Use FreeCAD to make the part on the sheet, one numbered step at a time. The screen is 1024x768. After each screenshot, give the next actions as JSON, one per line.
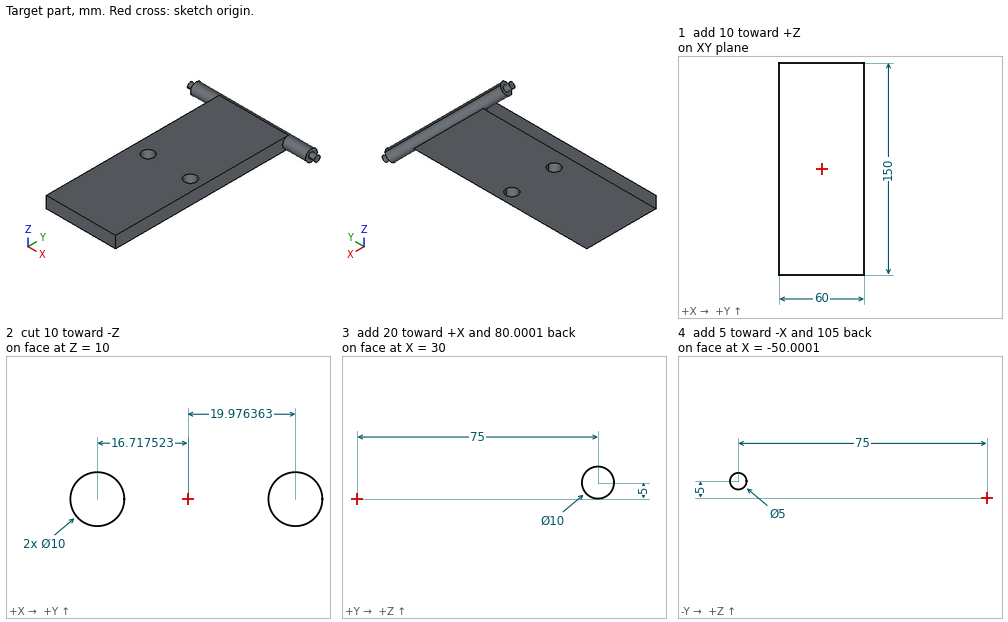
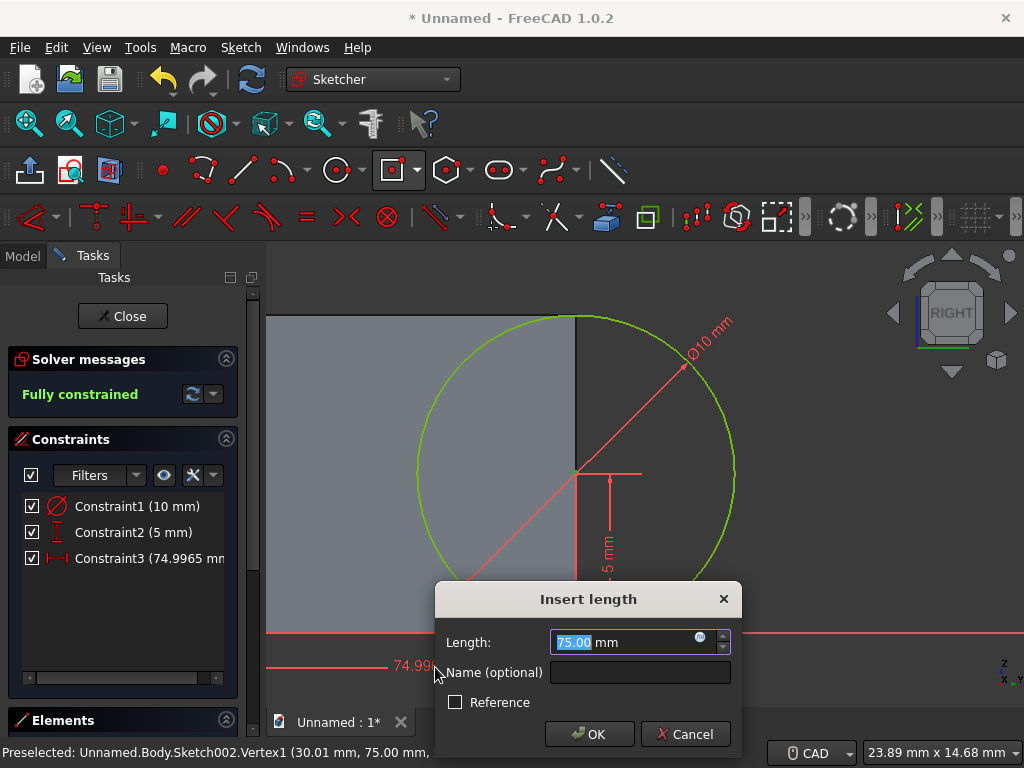
{"action": "type", "text": "75"}
{"action": "key", "text": "Return"}
{"action": "key", "text": "Escape"}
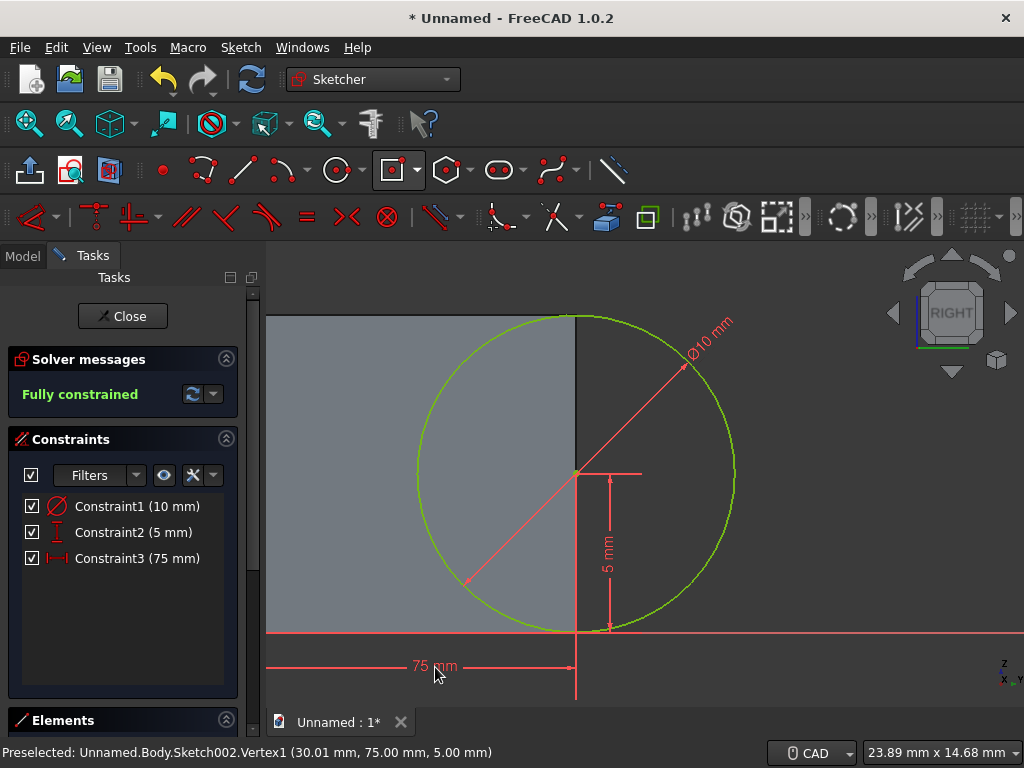
{"action": "left_click", "coordinate": [123, 316]}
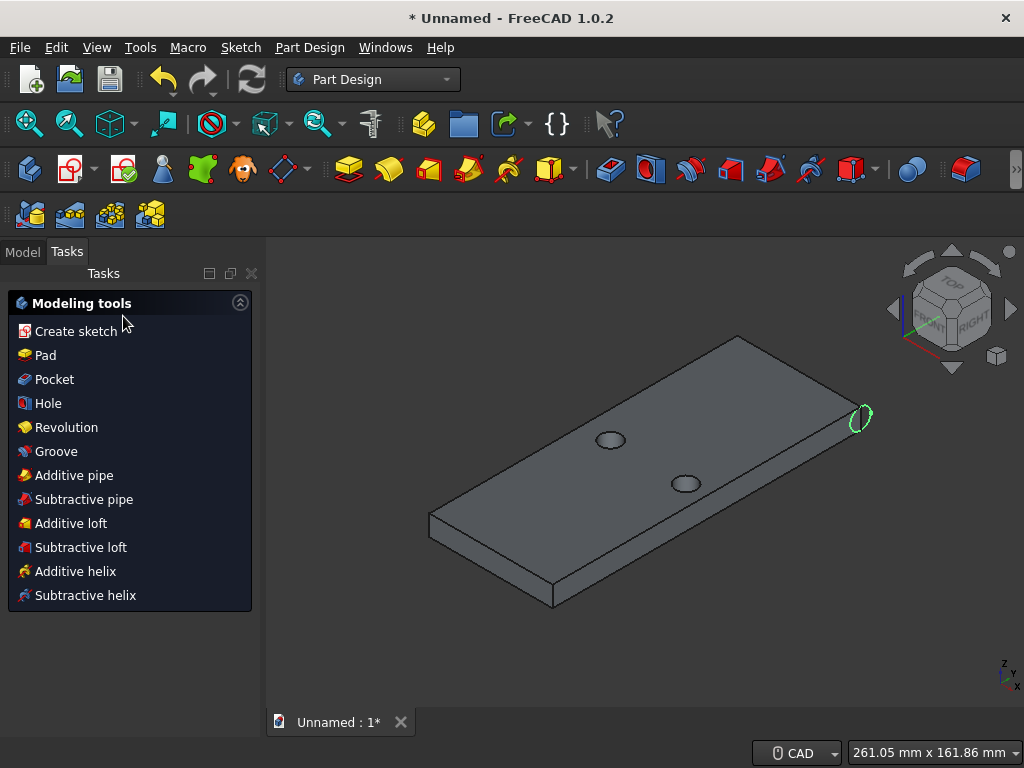
{"action": "left_click", "coordinate": [350, 170]}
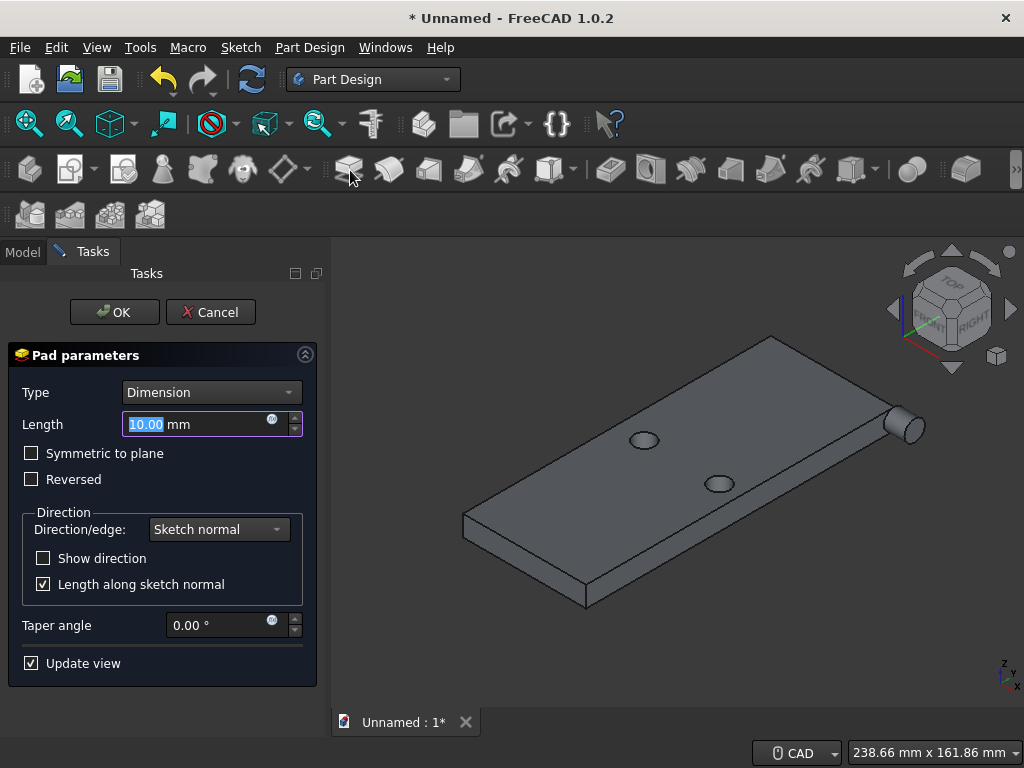
{"action": "left_click", "coordinate": [212, 392]}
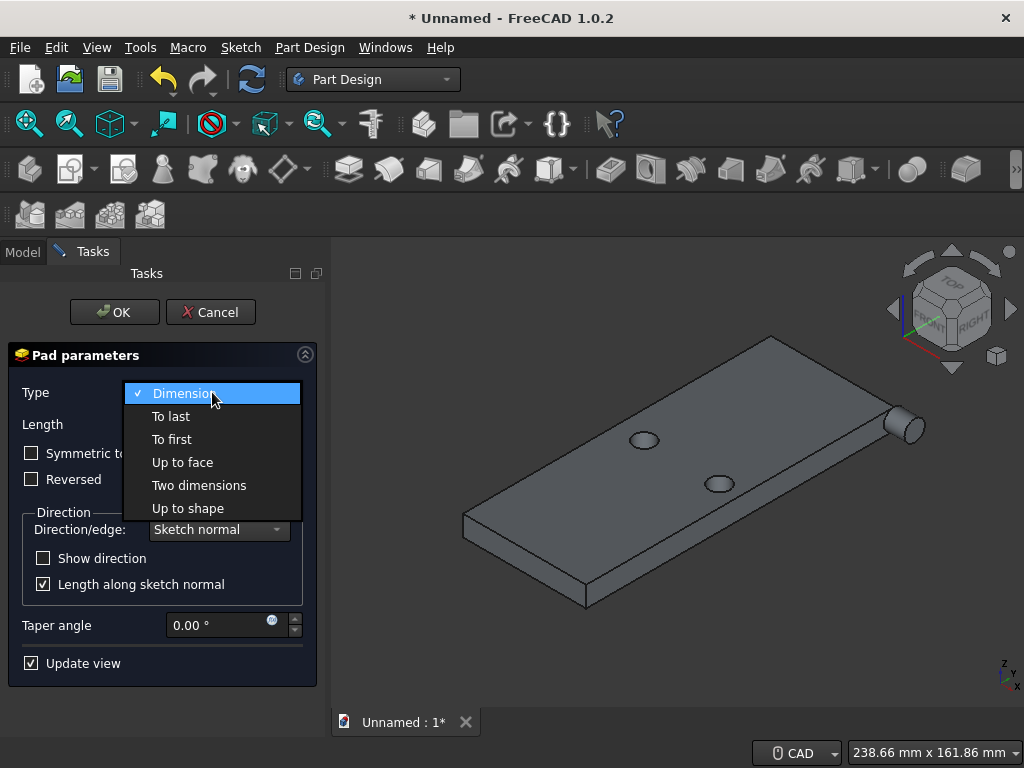
{"action": "left_click", "coordinate": [212, 486]}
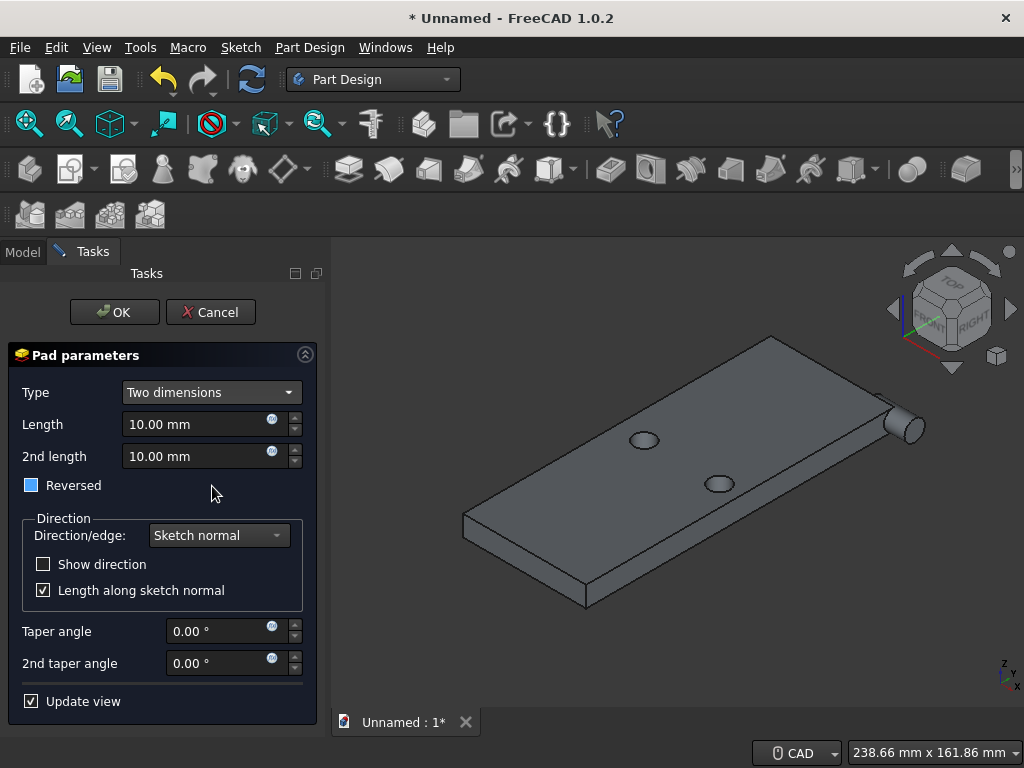
{"action": "triple_click", "coordinate": [204, 424]}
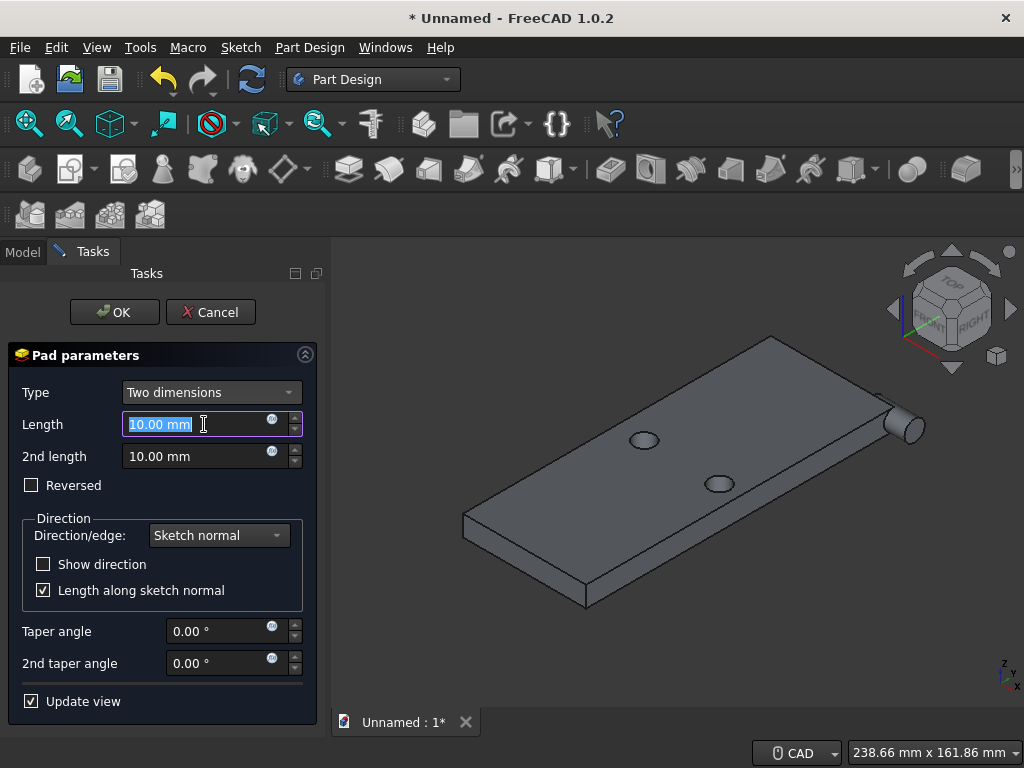
{"action": "type", "text": "20"}
{"action": "key", "text": "Tab"}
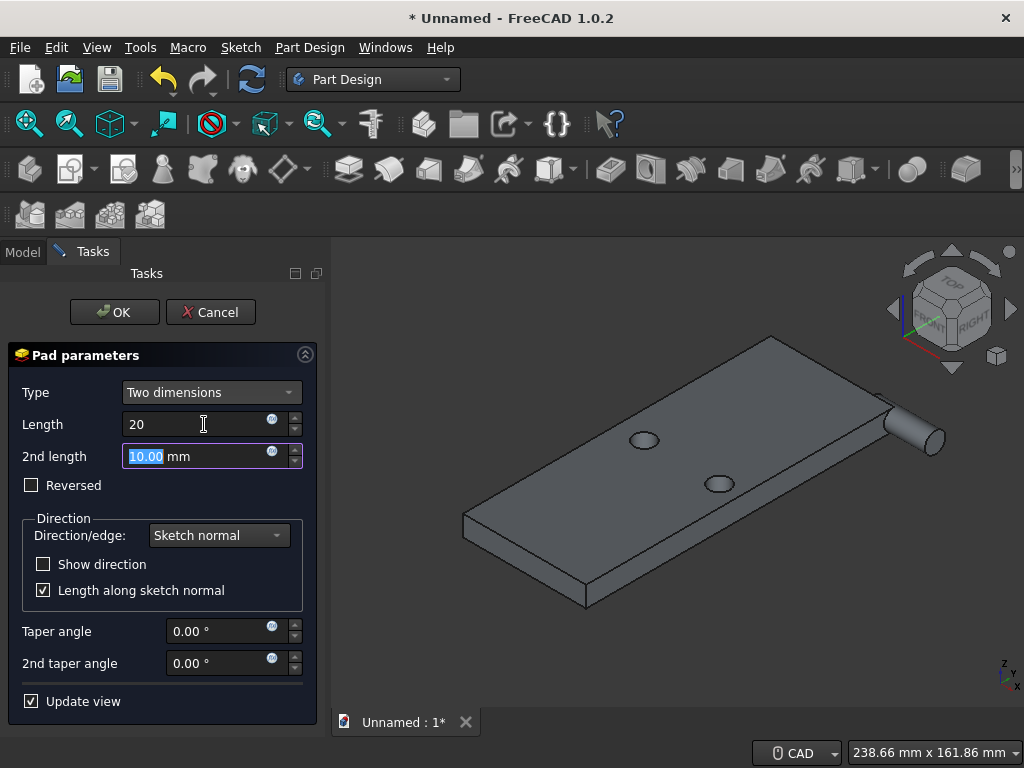
{"action": "type", "text": "80.0001"}
{"action": "key", "text": "Tab"}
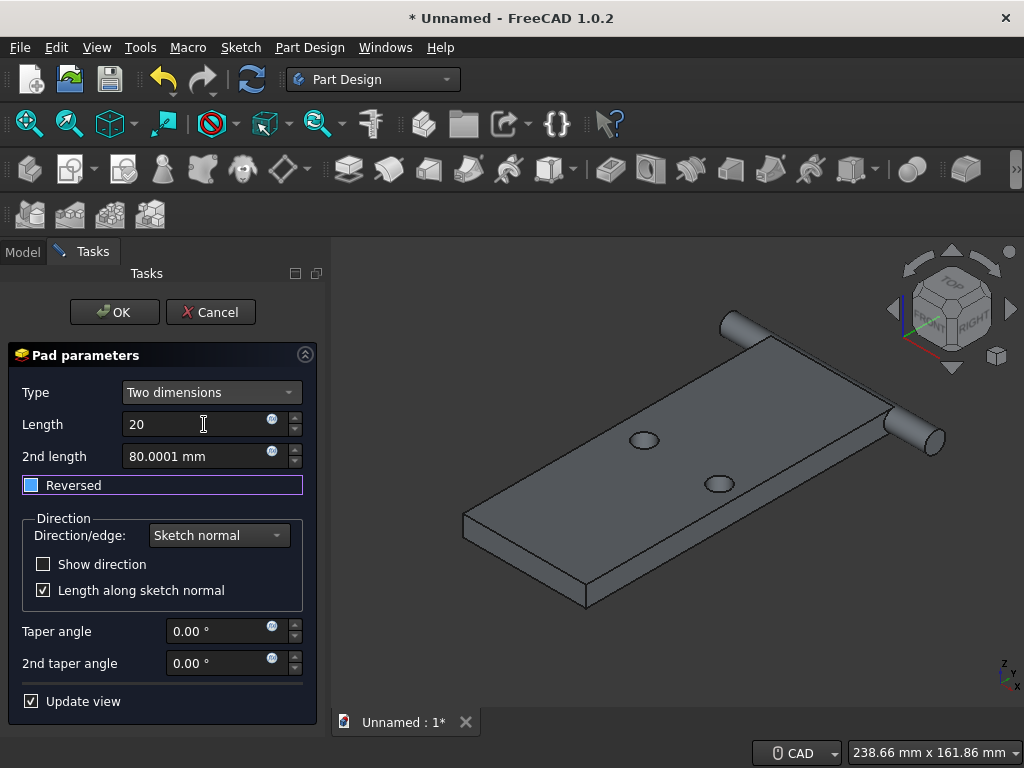
{"action": "left_click", "coordinate": [115, 312]}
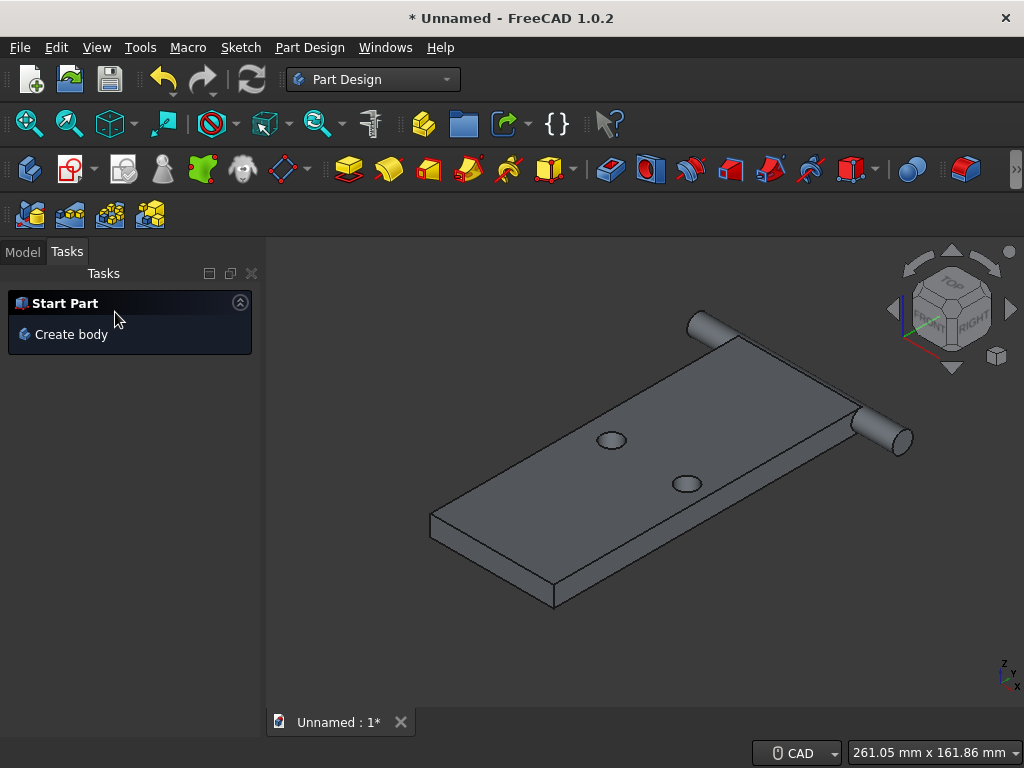
{"action": "key", "text": "6"}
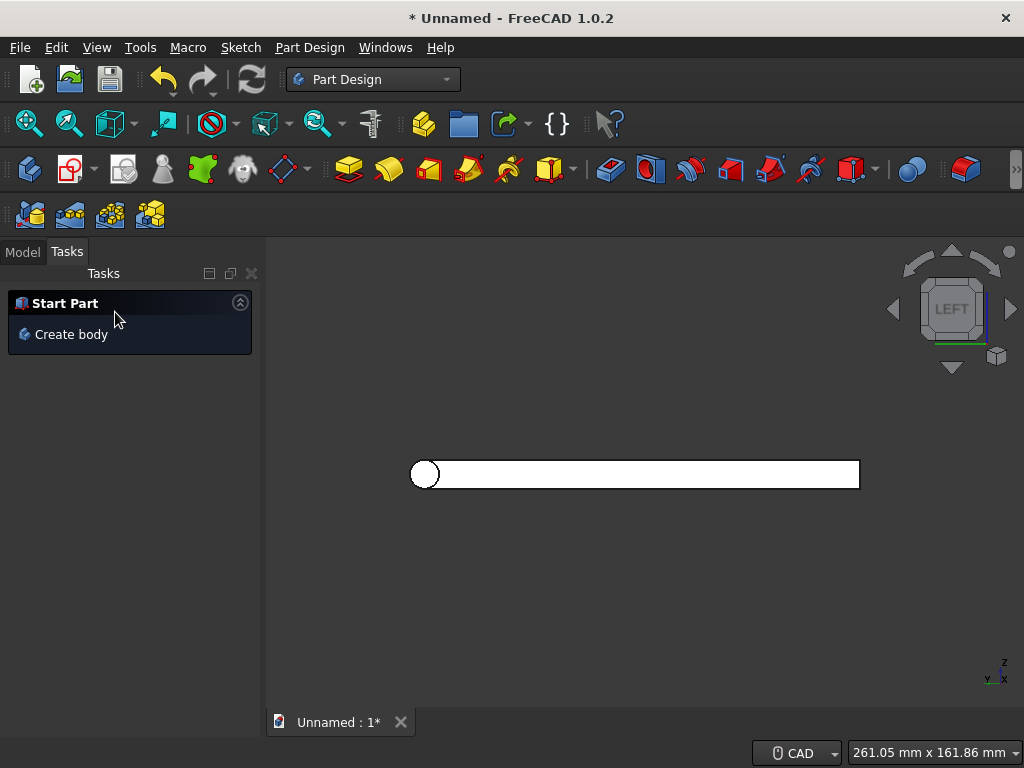
{"action": "left_click", "coordinate": [424, 473]}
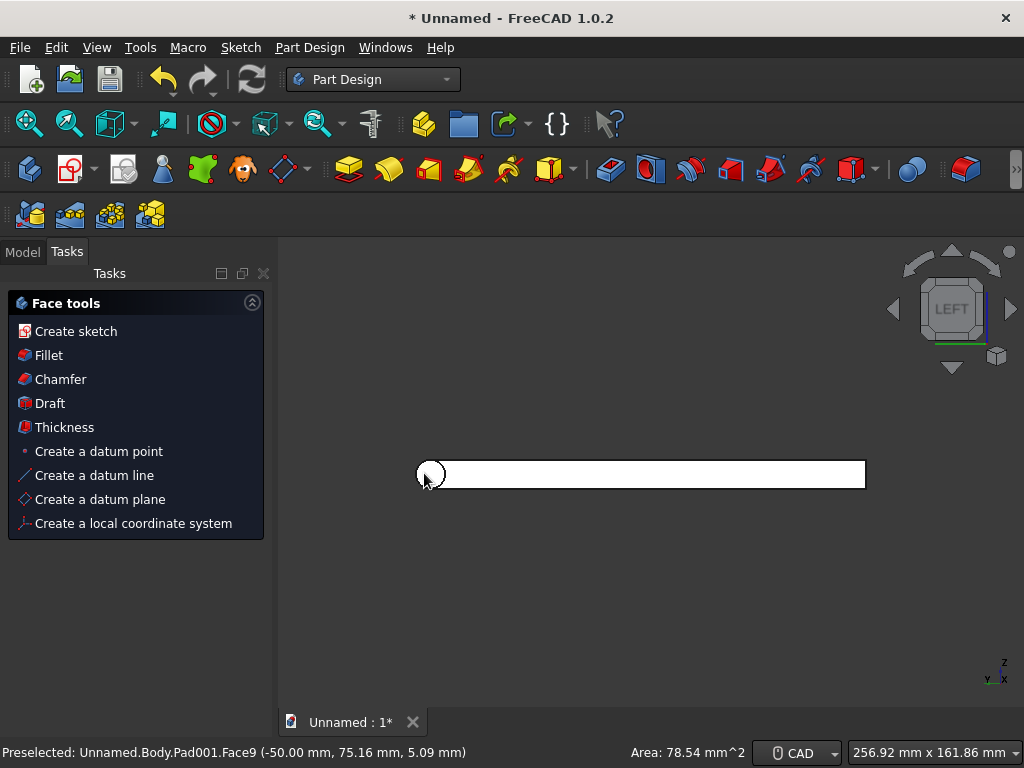
{"action": "left_click", "coordinate": [70, 170]}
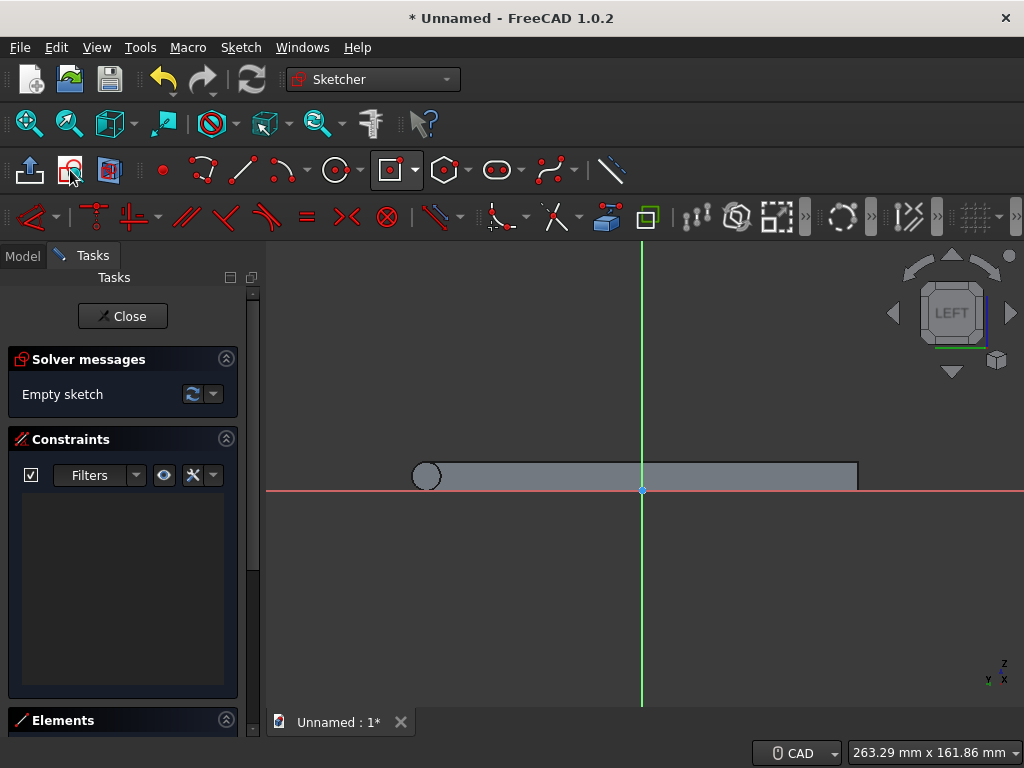
{"action": "scroll", "coordinate": [418, 476], "scroll_direction": "up", "scroll_amount": 15}